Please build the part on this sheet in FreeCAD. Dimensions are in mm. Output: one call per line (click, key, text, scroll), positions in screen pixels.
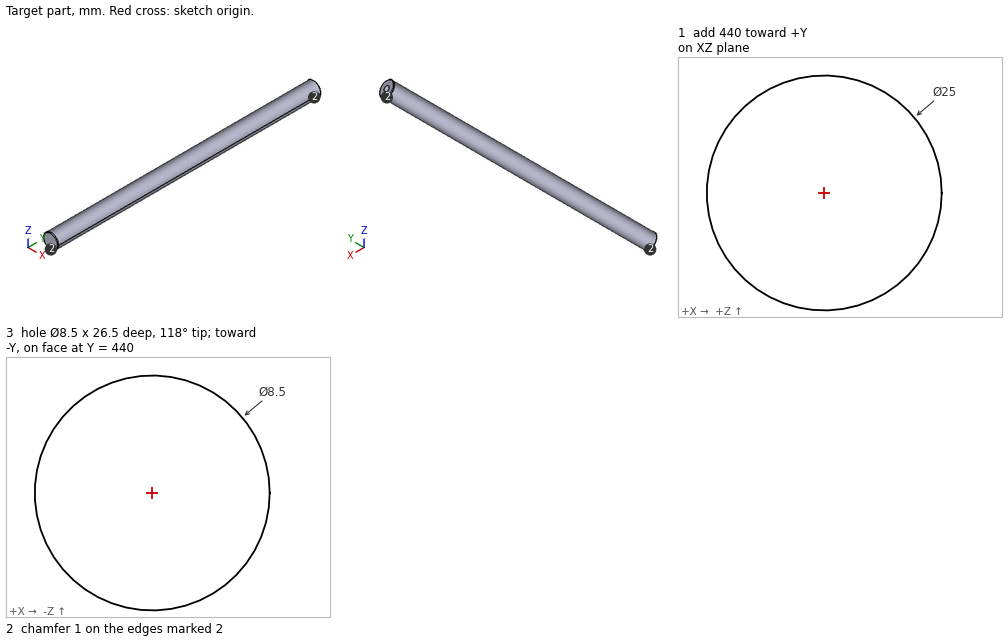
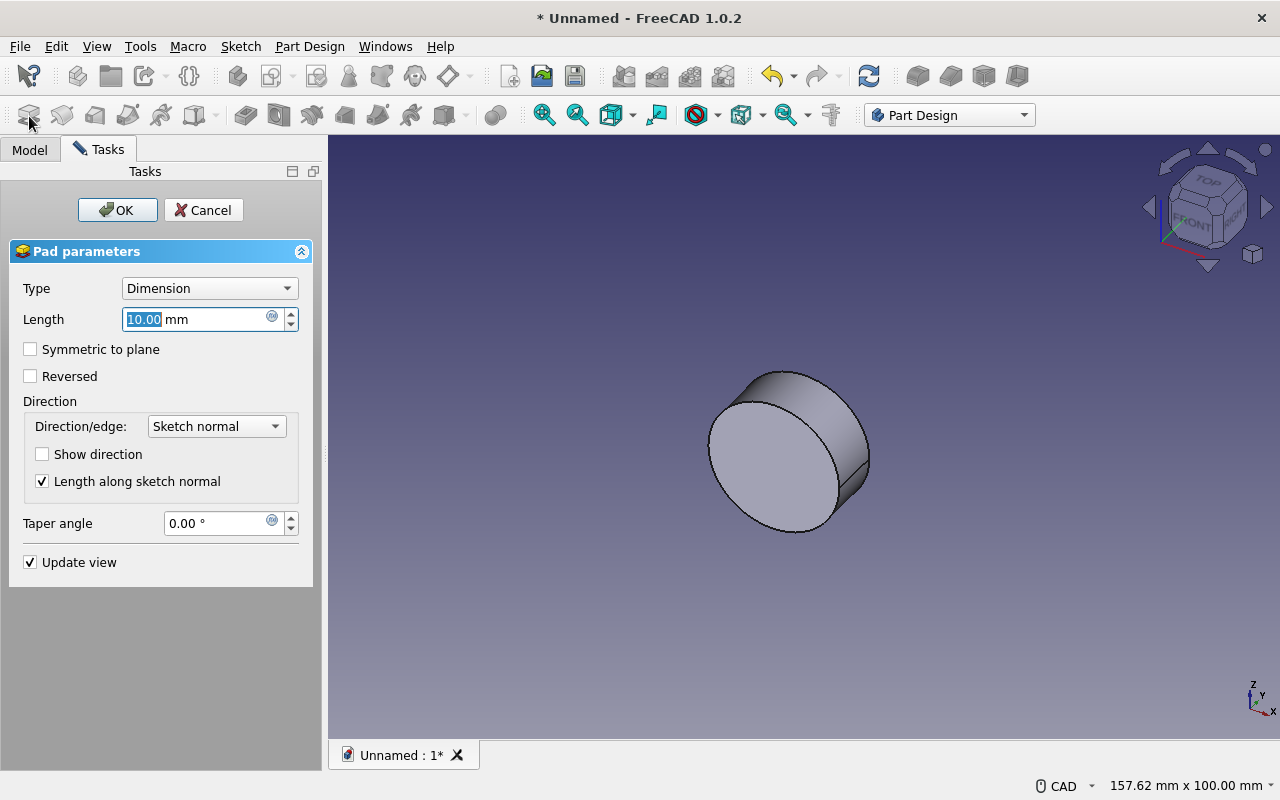
text(440)
key(Tab)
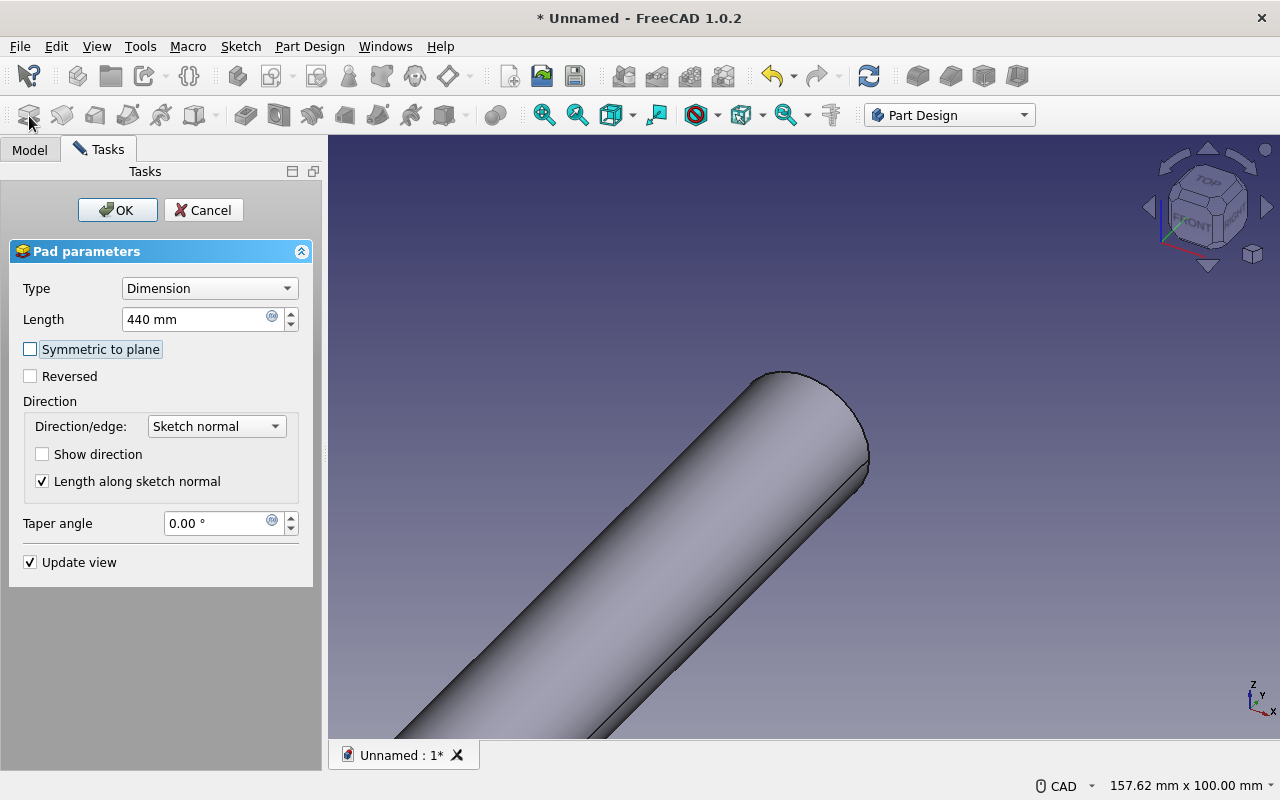
click(31, 376)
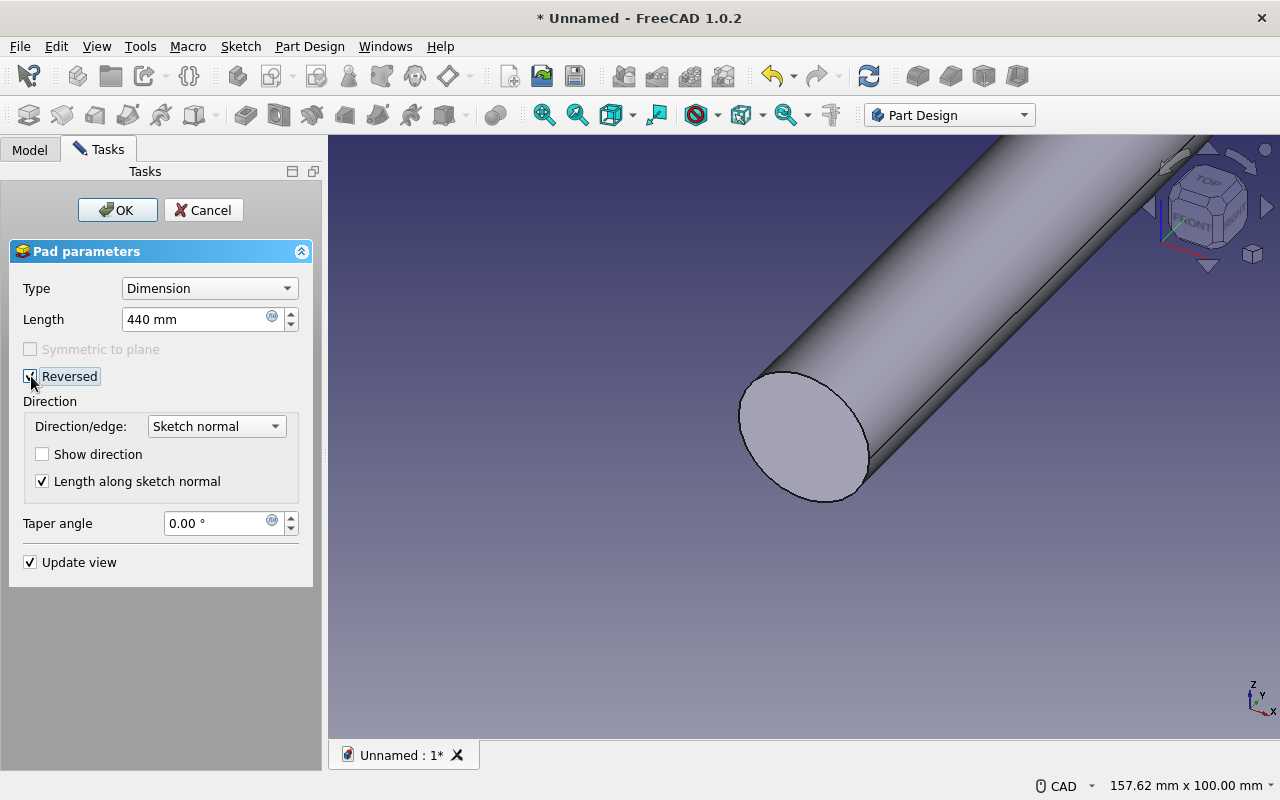
click(118, 210)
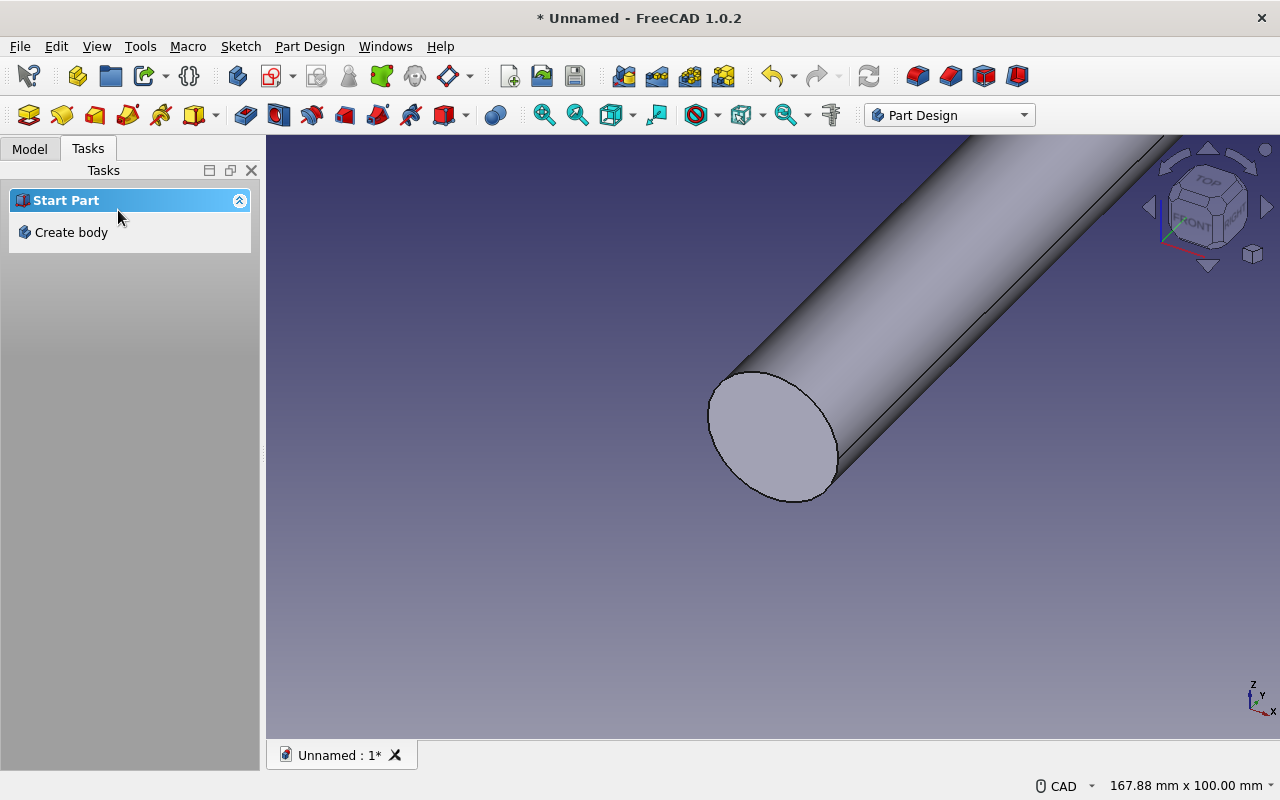
click(545, 116)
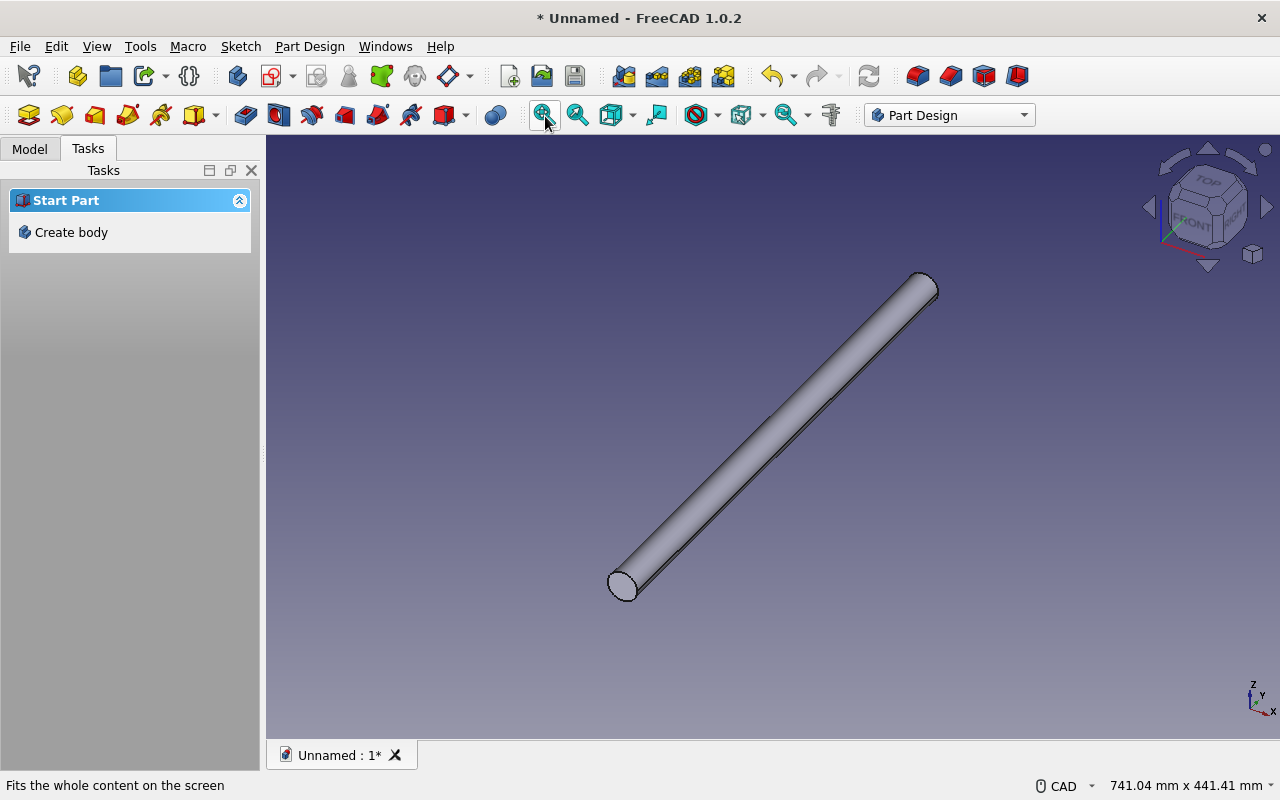
click(608, 581)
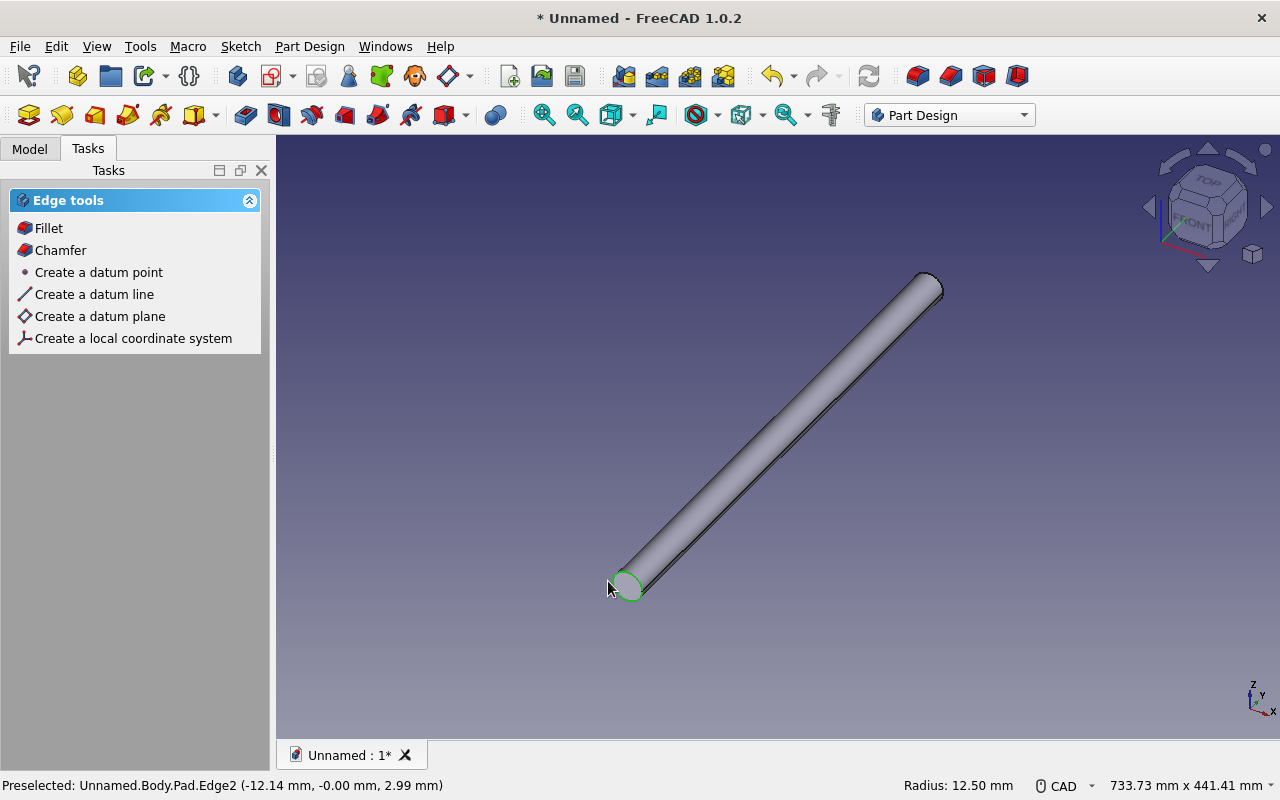
key(0)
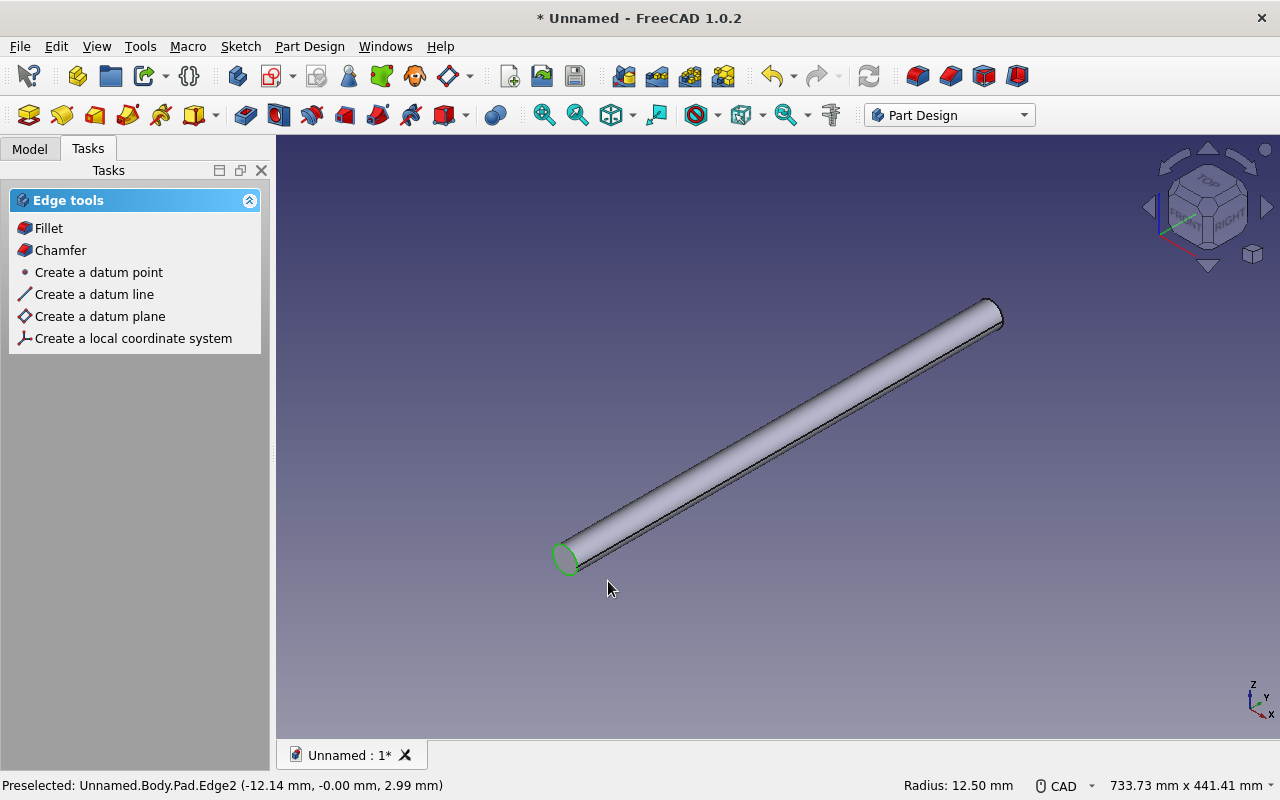
click(987, 298, ctrl)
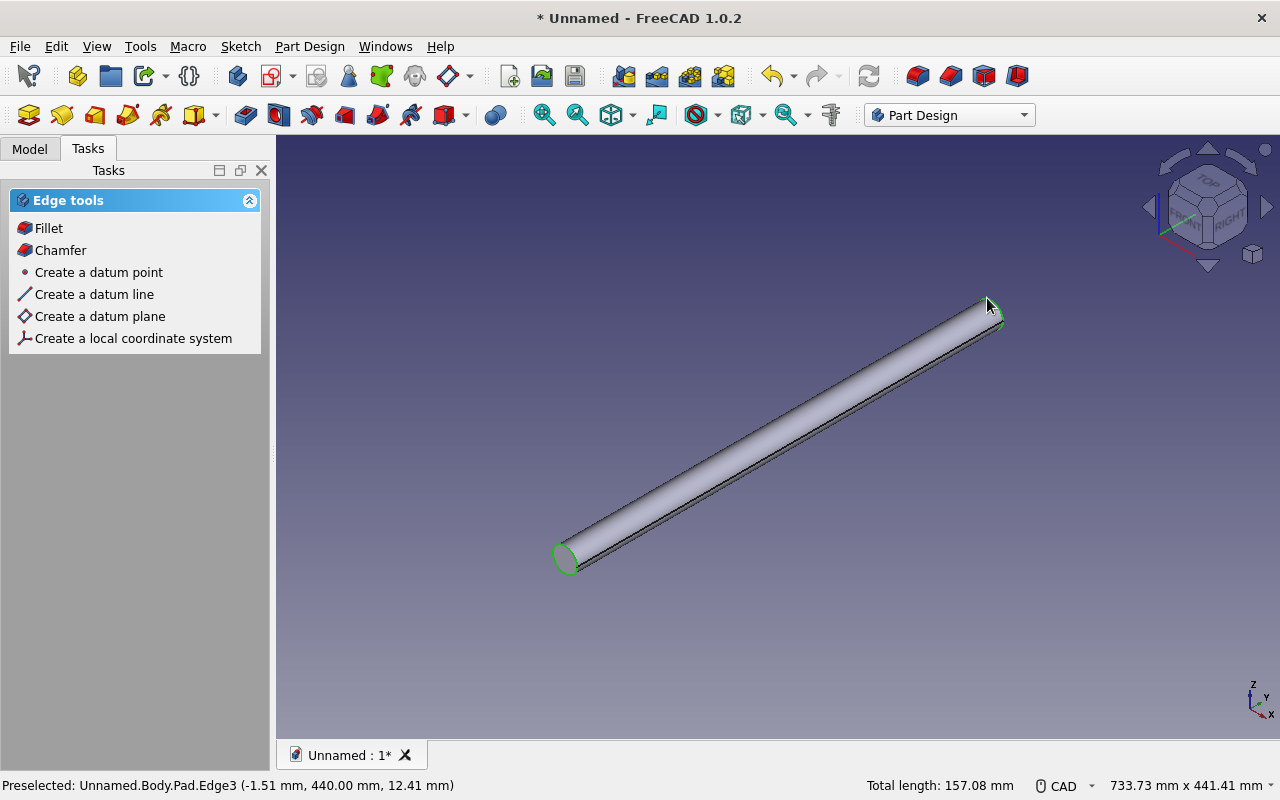
click(951, 76)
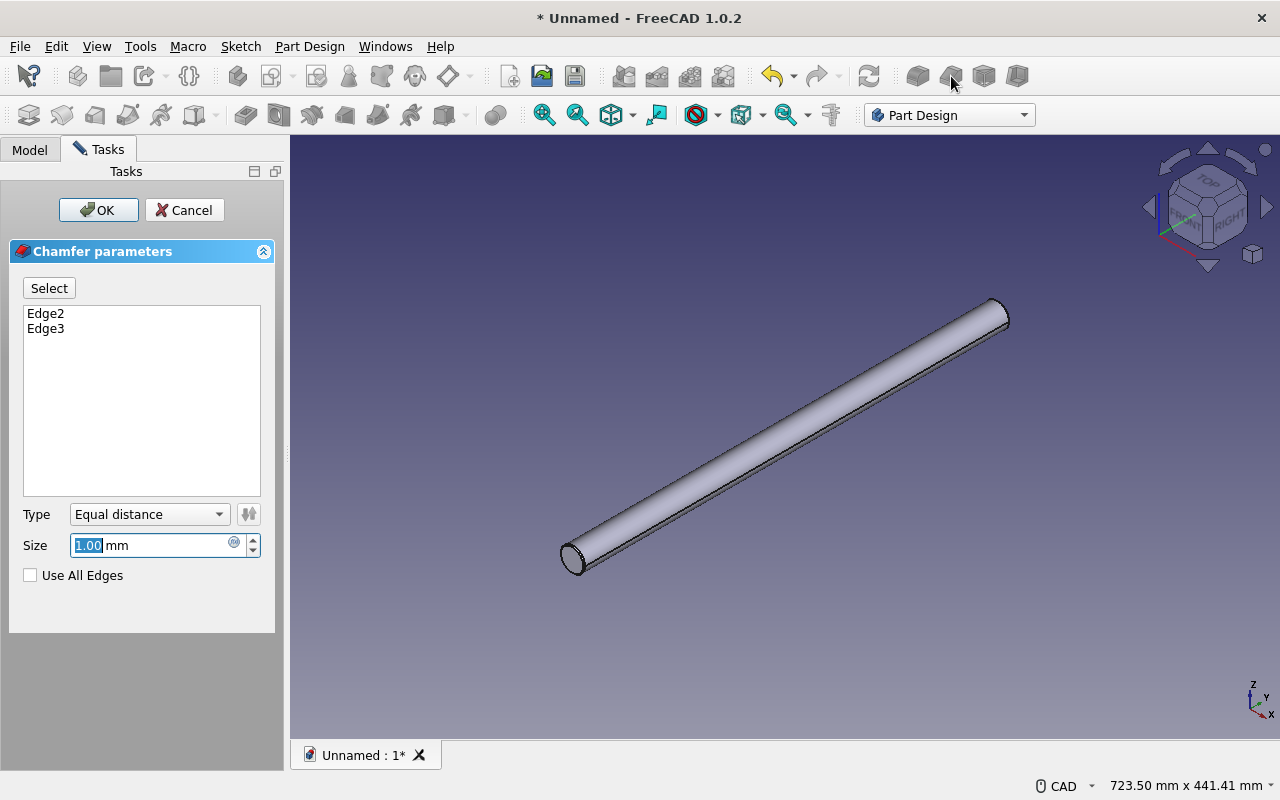
text(1)
key(Tab)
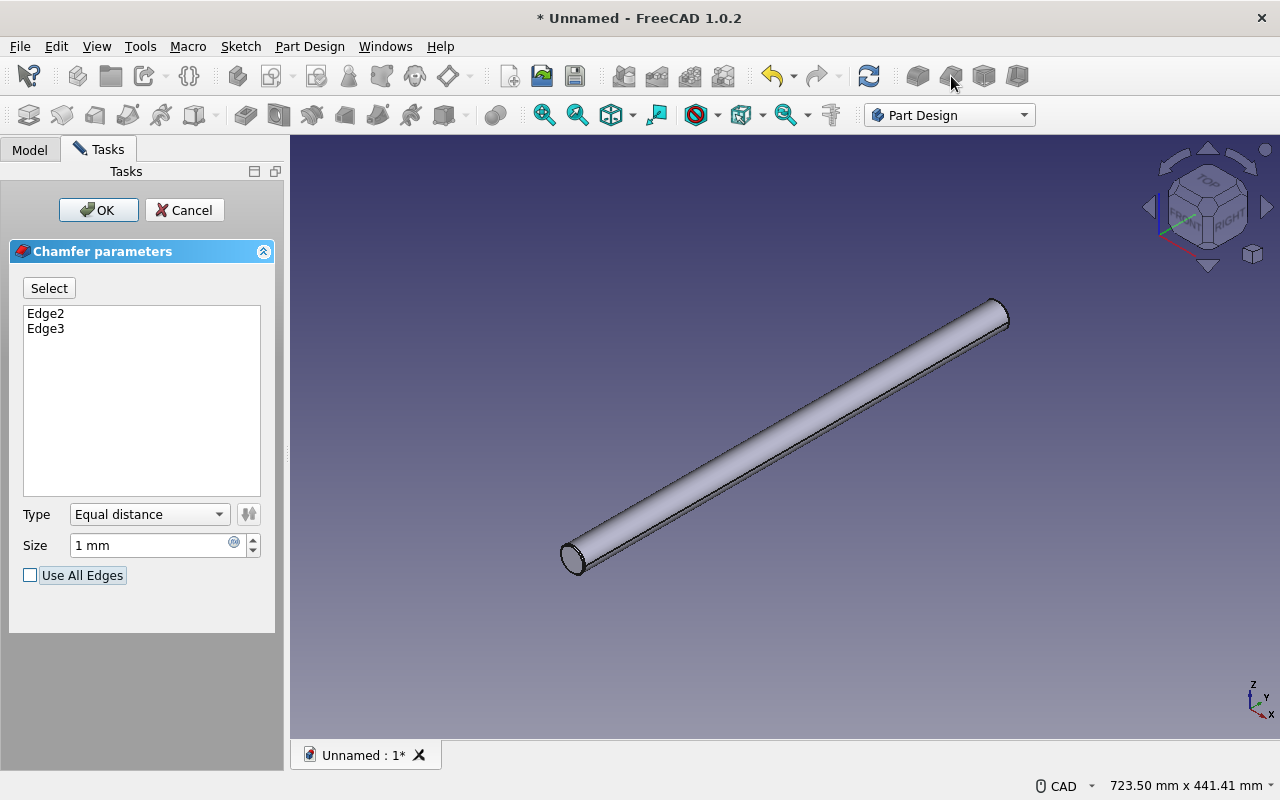
click(99, 210)